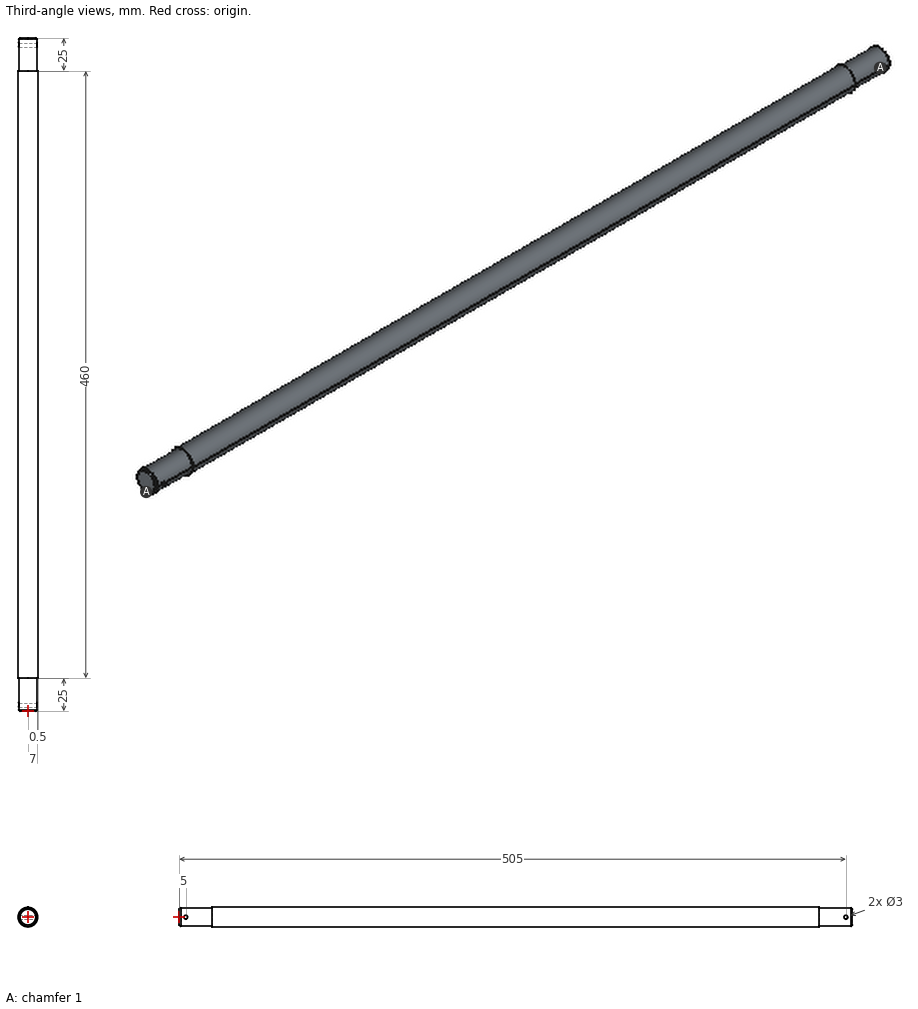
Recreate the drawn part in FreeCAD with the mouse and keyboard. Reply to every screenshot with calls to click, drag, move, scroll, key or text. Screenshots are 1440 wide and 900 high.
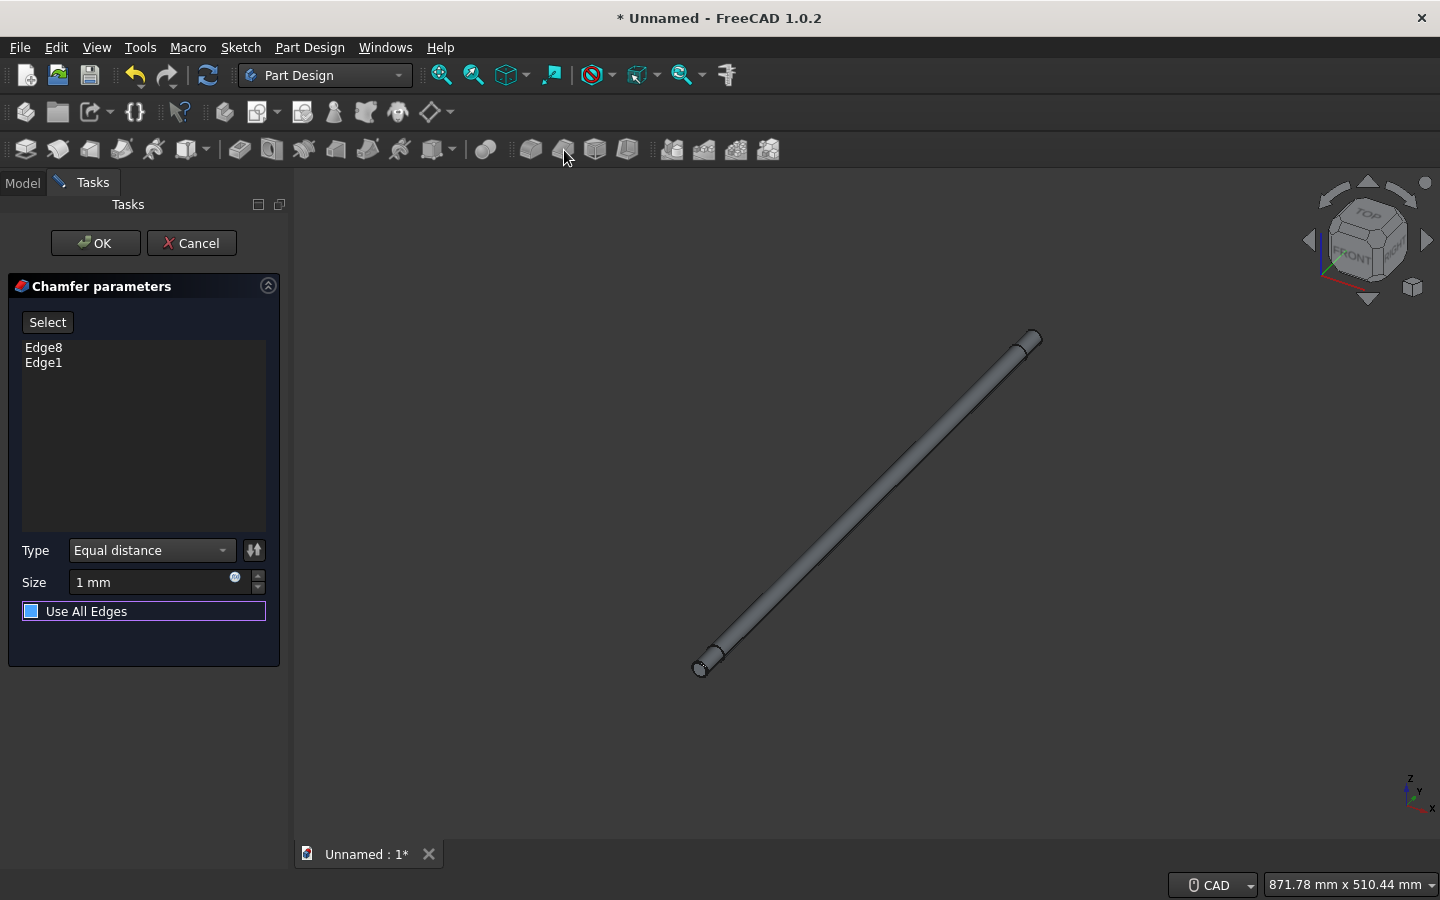
click(96, 243)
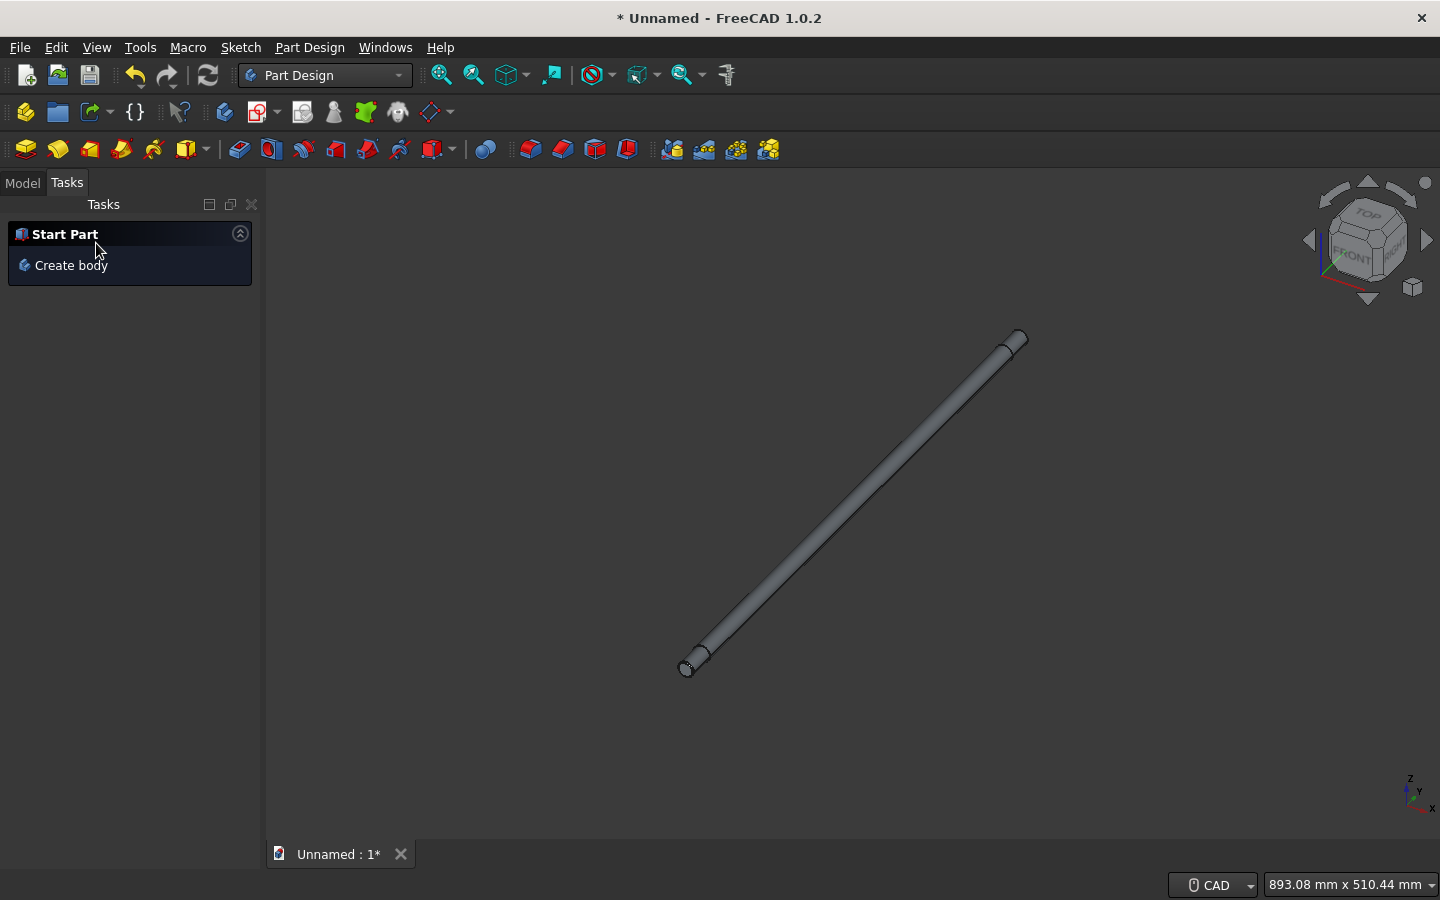
click(258, 112)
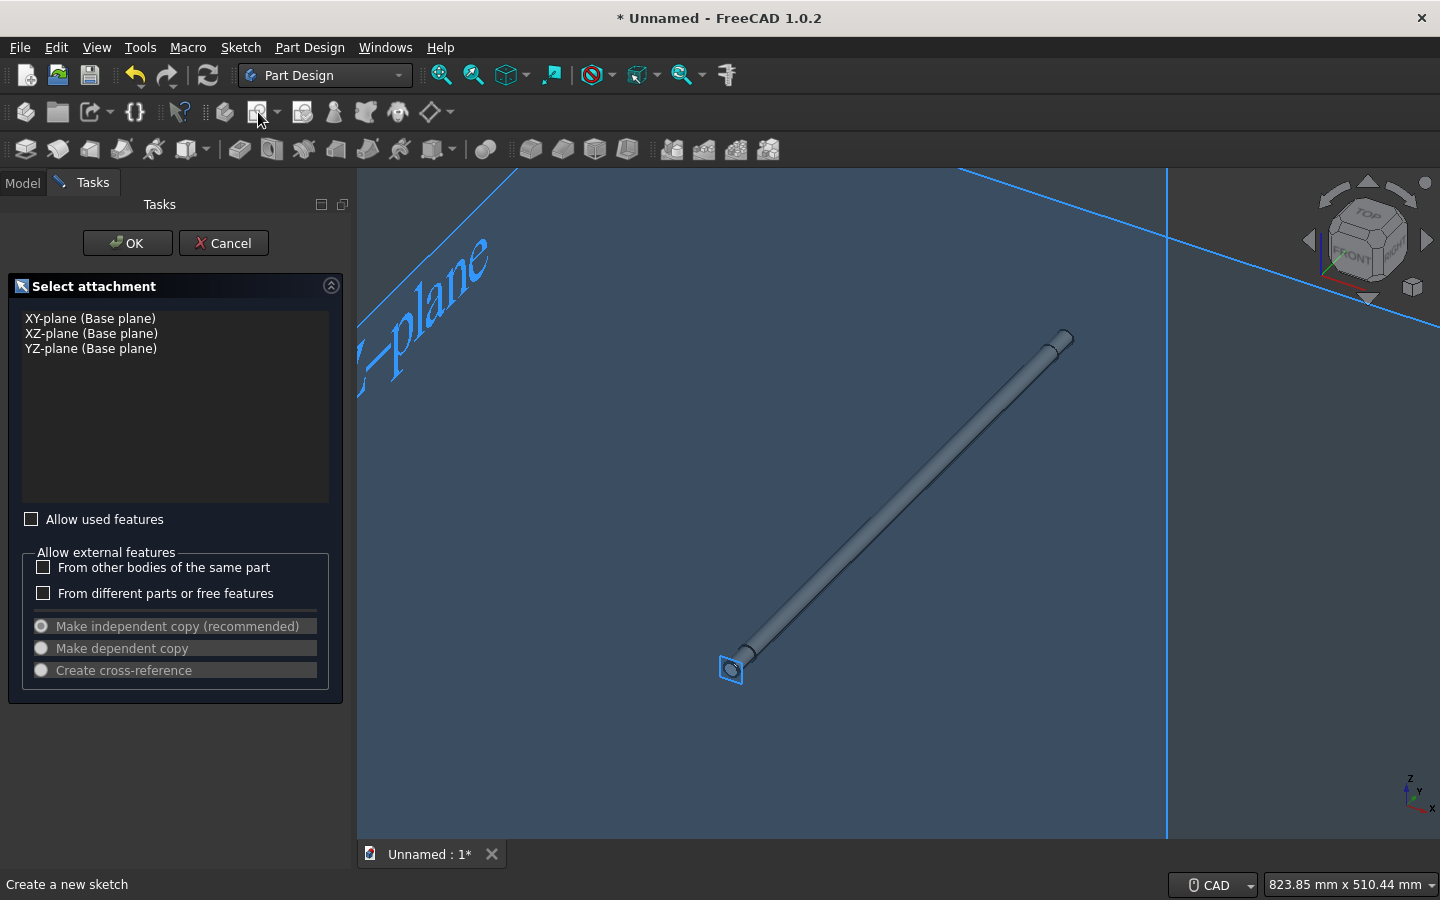
click(82, 348)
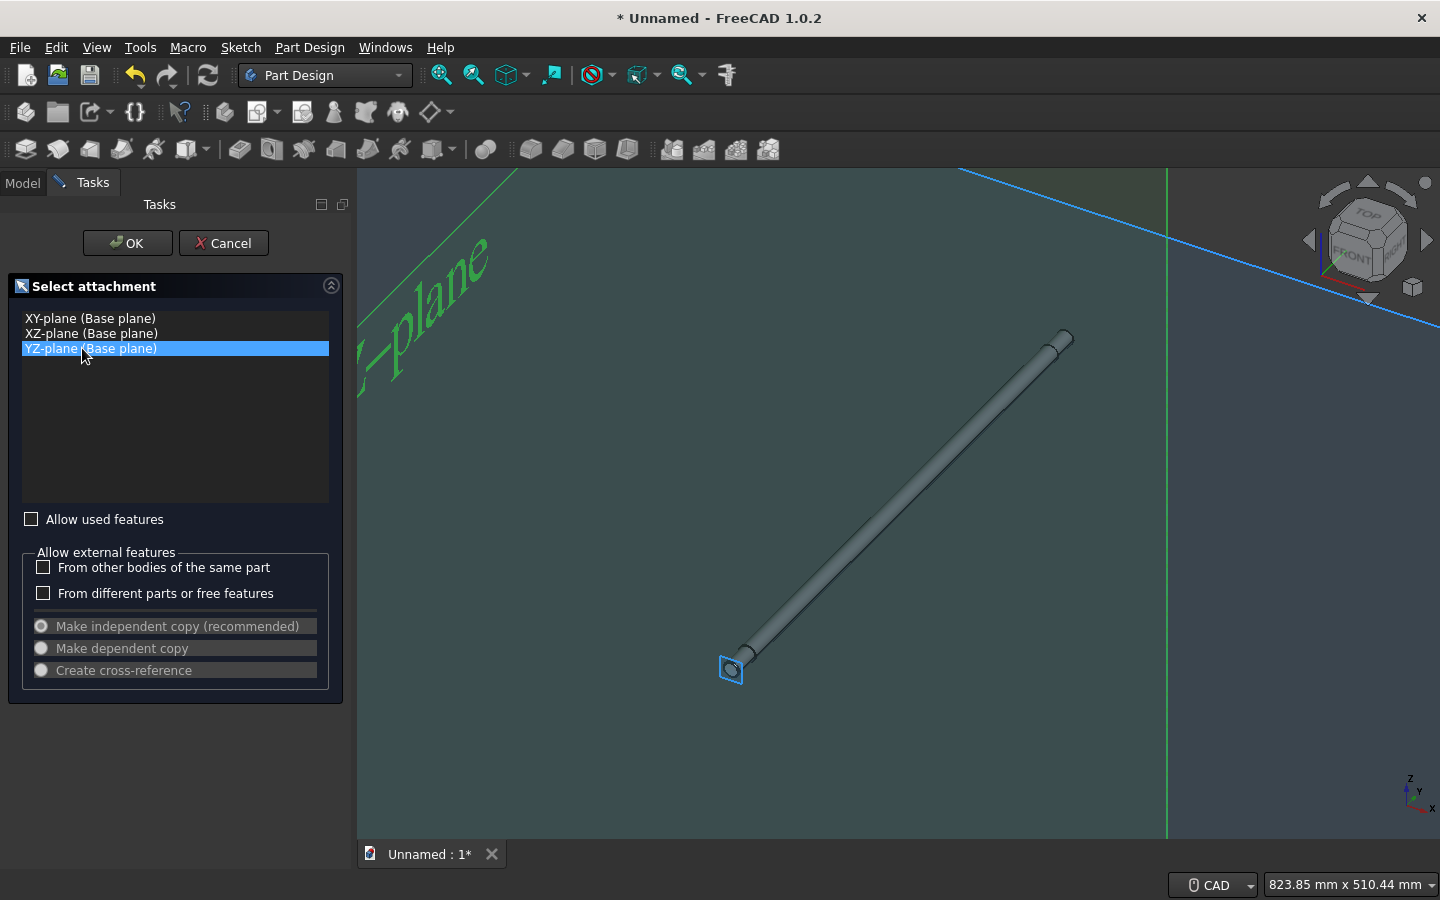
click(128, 243)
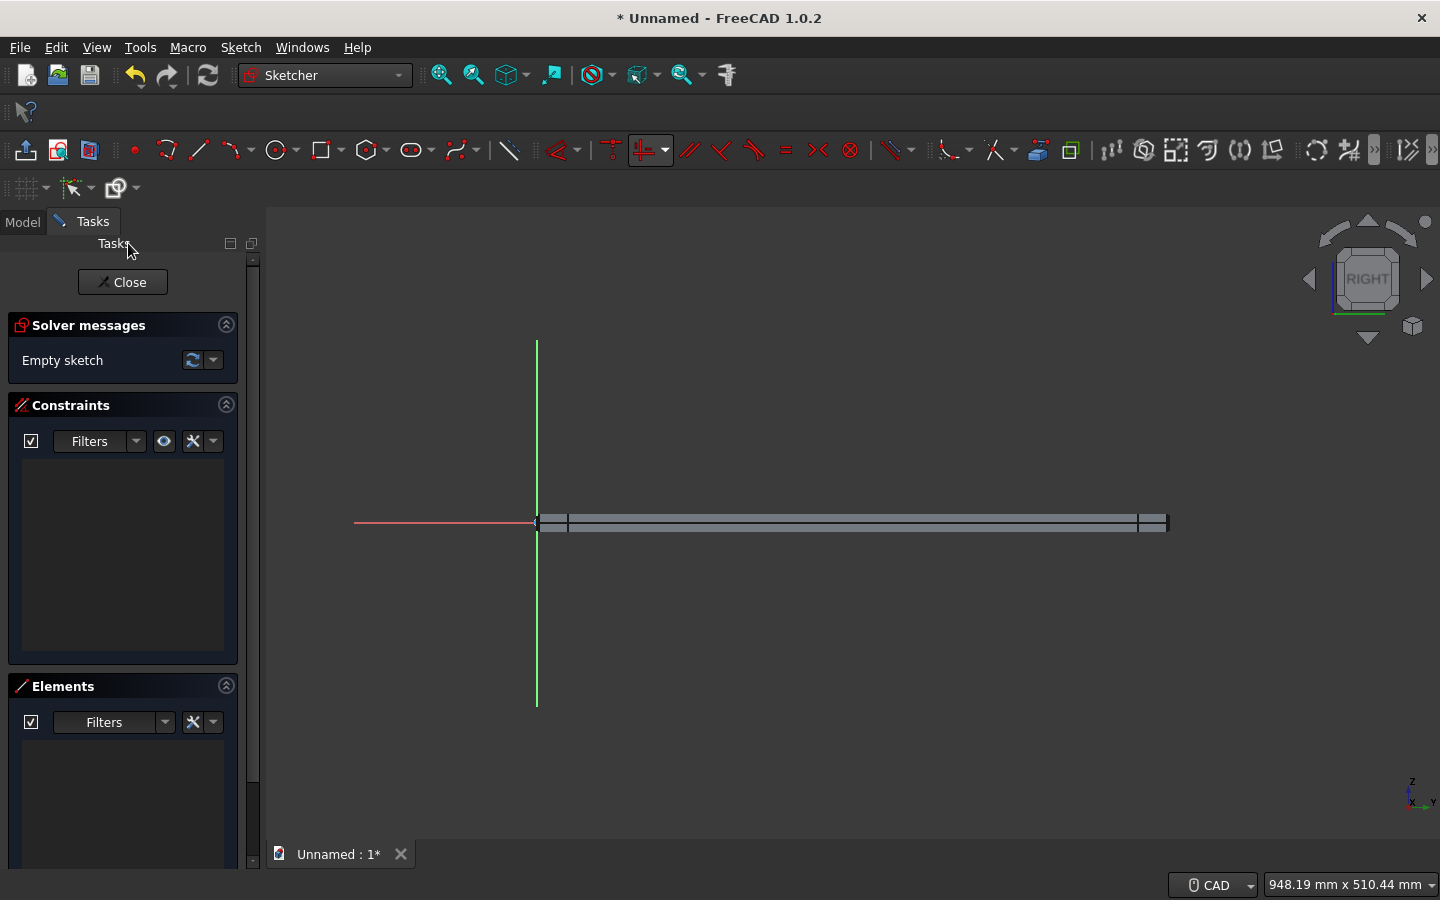
click(90, 150)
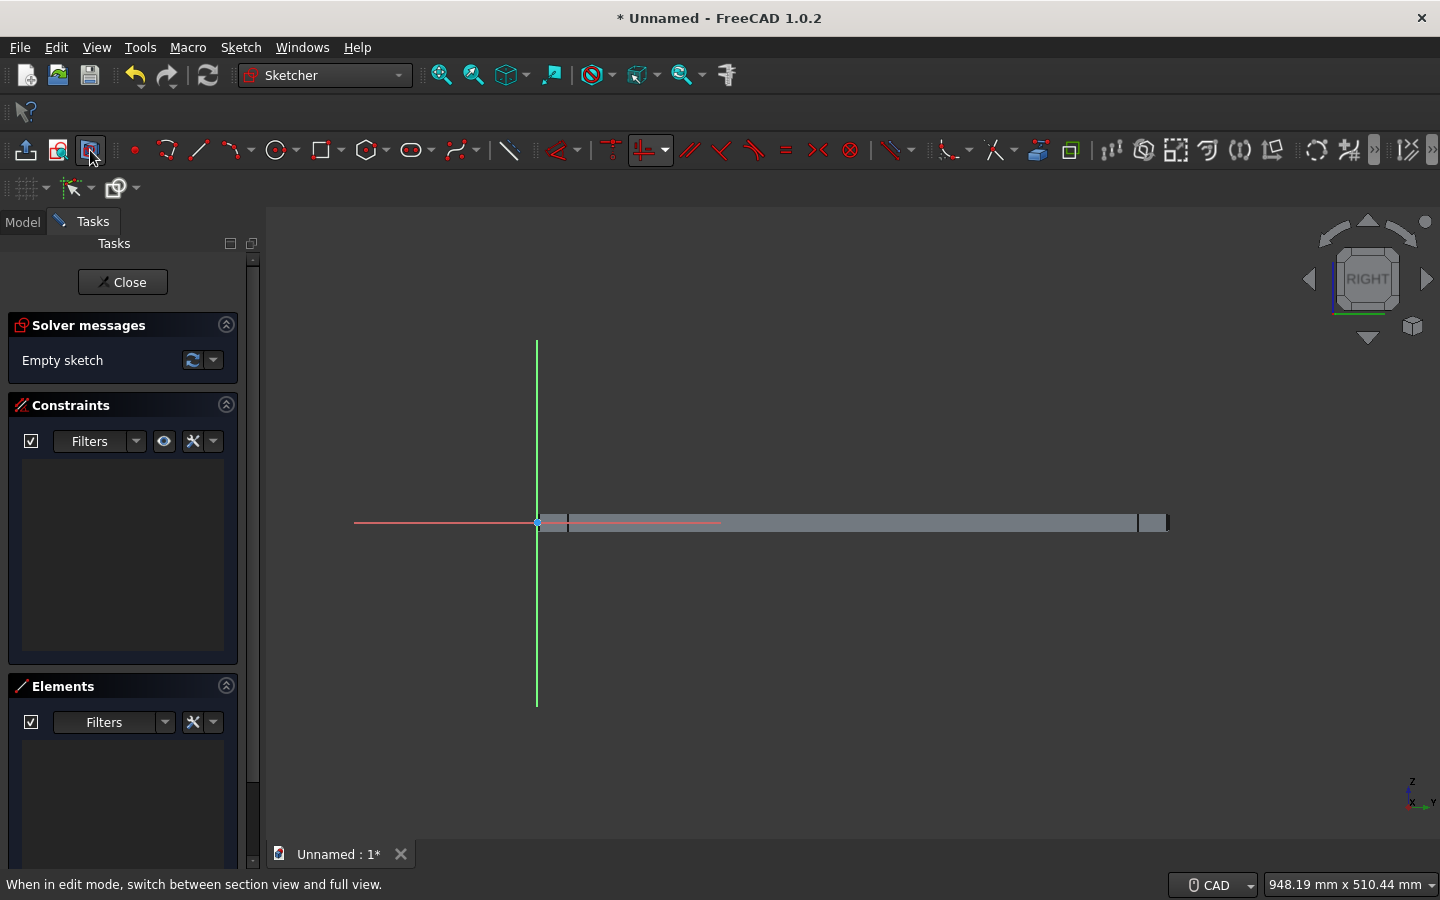
click(276, 150)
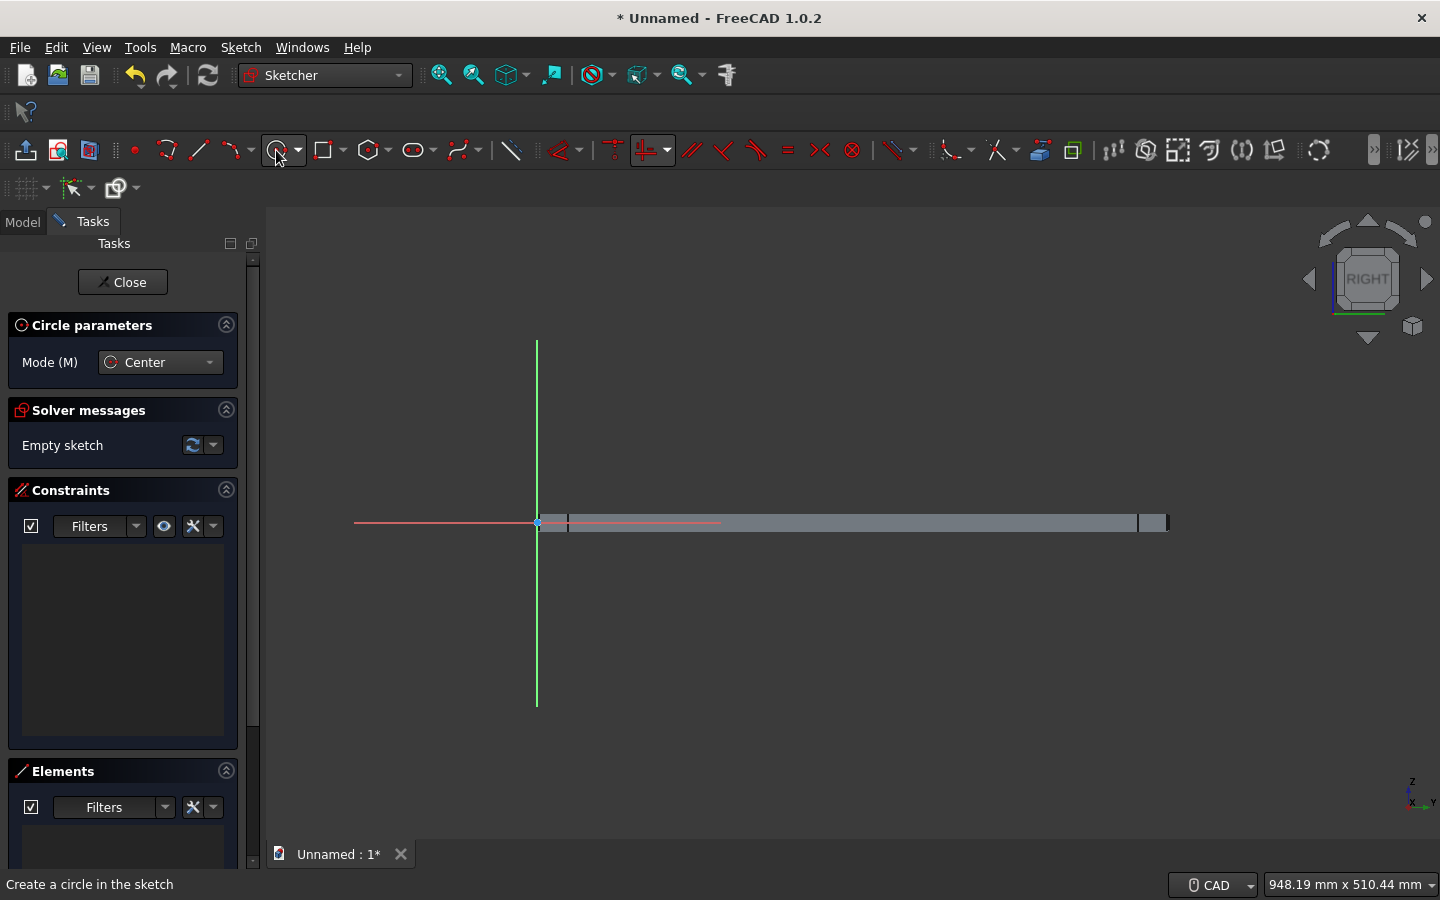
scroll(1163, 523, up, 13)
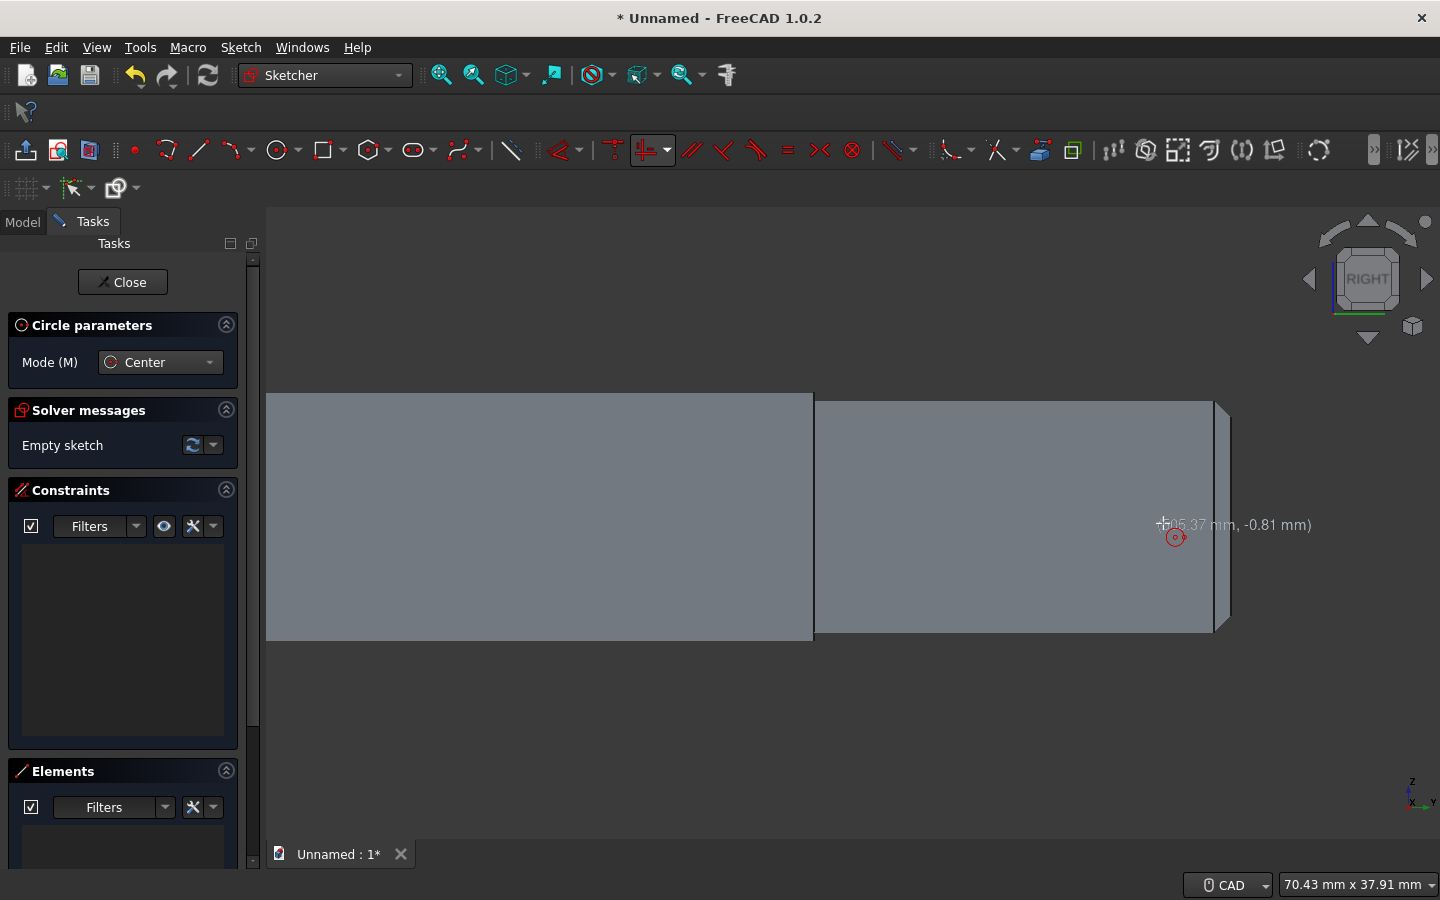
scroll(1092, 524, down, 13)